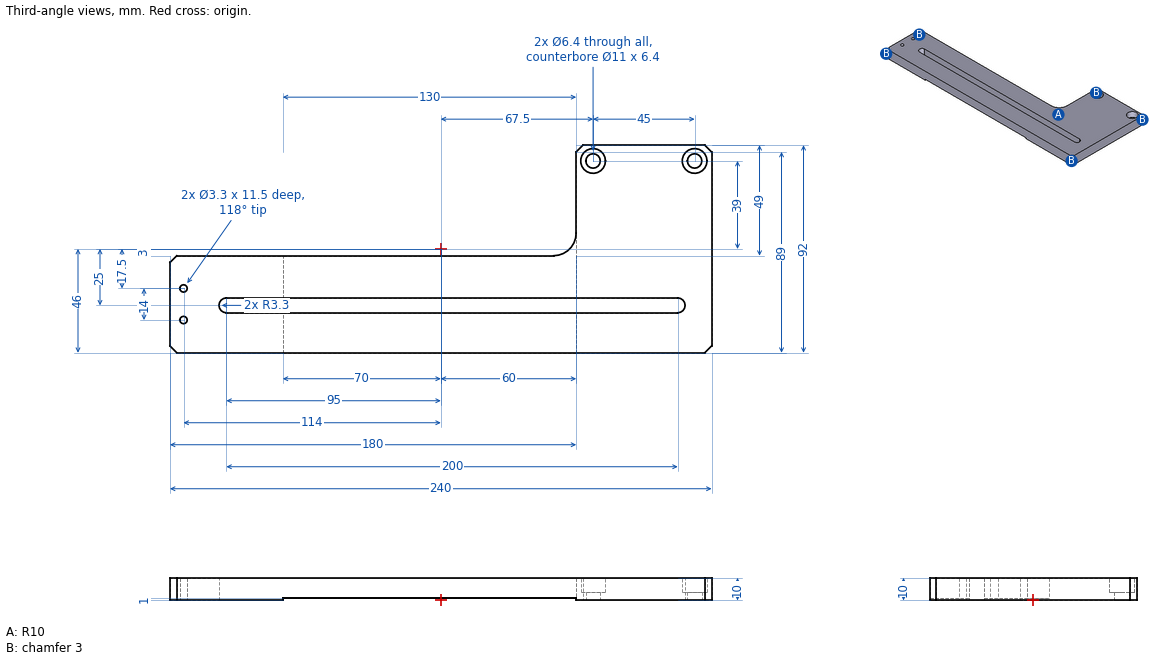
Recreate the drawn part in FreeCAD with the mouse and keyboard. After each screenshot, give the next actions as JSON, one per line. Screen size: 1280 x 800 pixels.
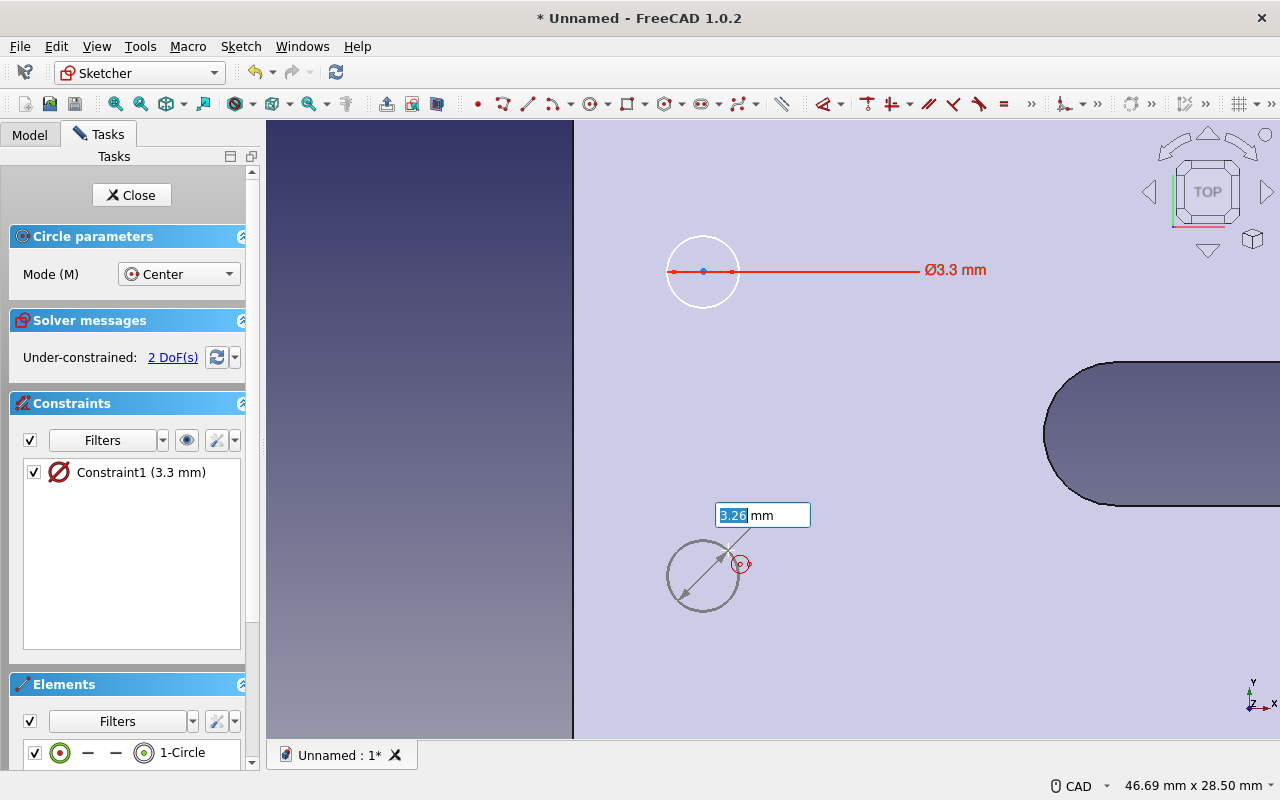
{"action": "type", "text": "3.3"}
{"action": "key", "text": "Return"}
{"action": "key", "text": "Escape"}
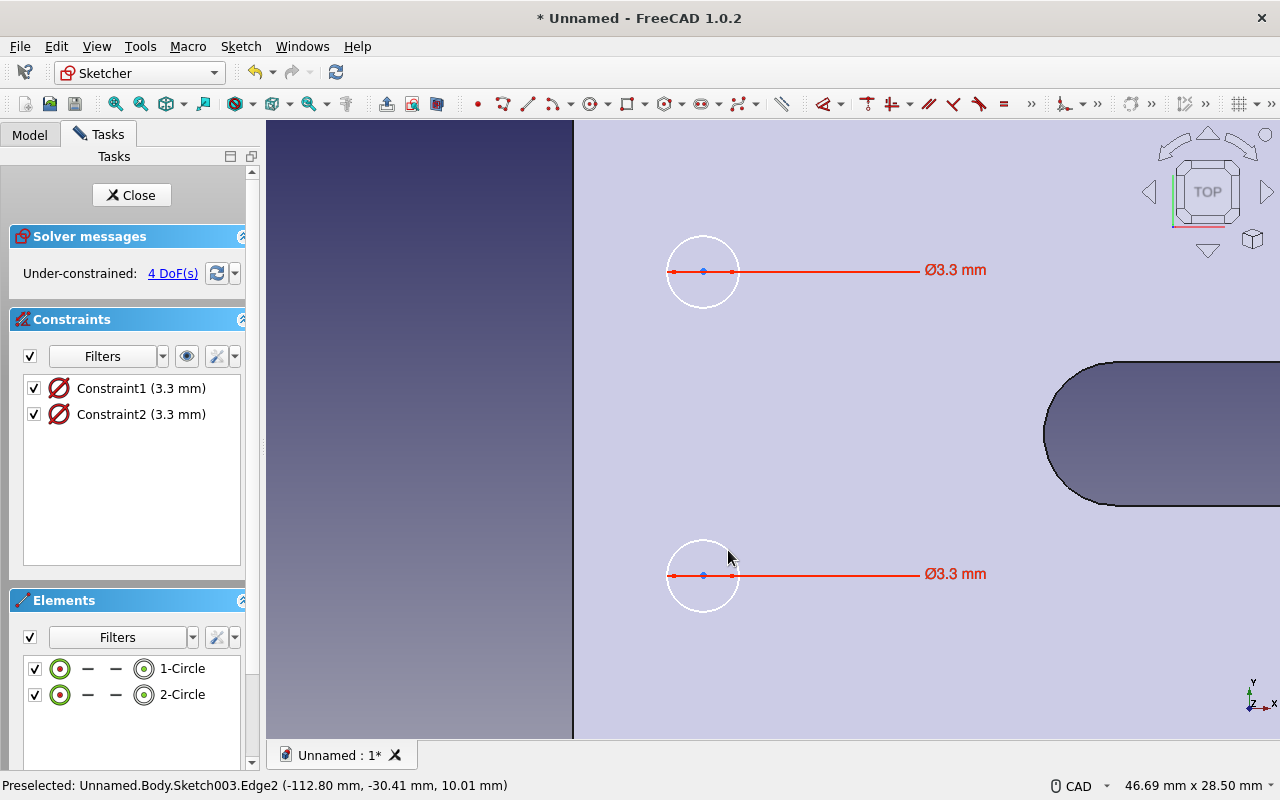
{"action": "left_click", "coordinate": [703, 272]}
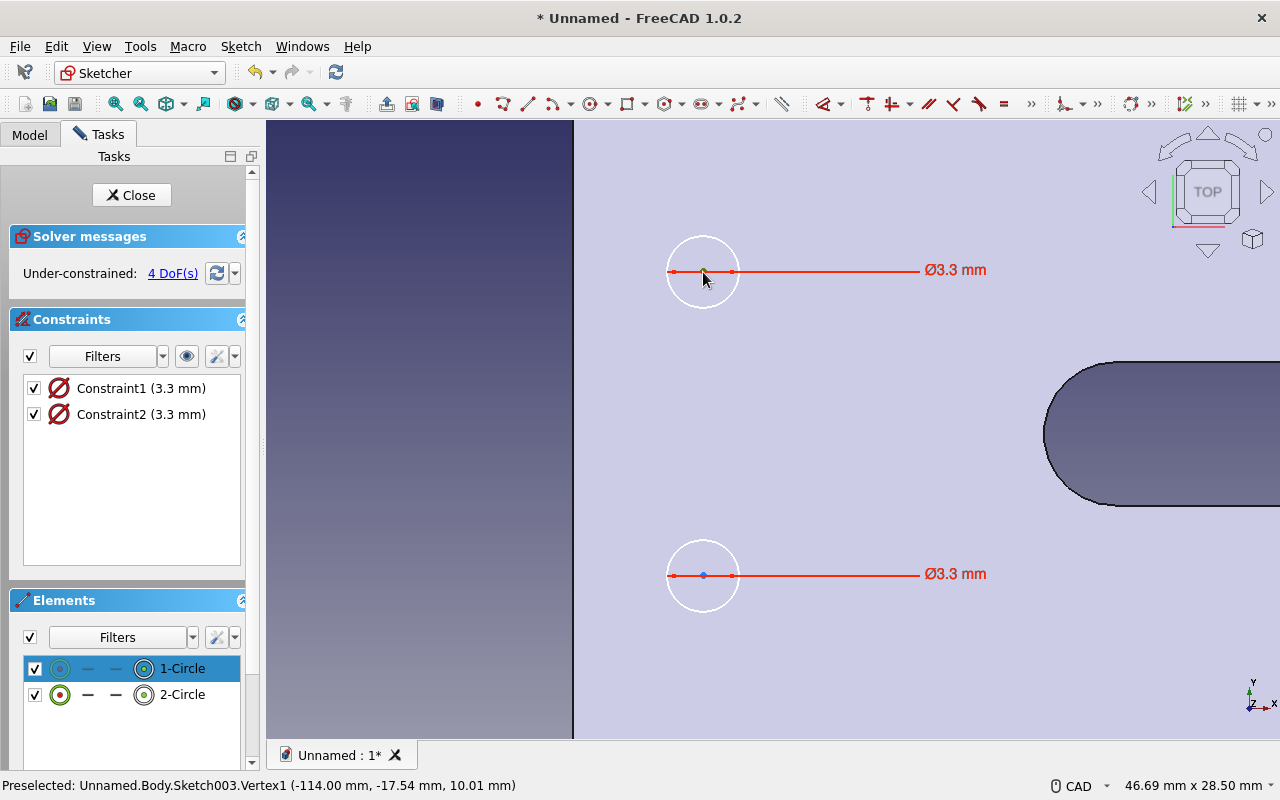
{"action": "left_click", "coordinate": [840, 104]}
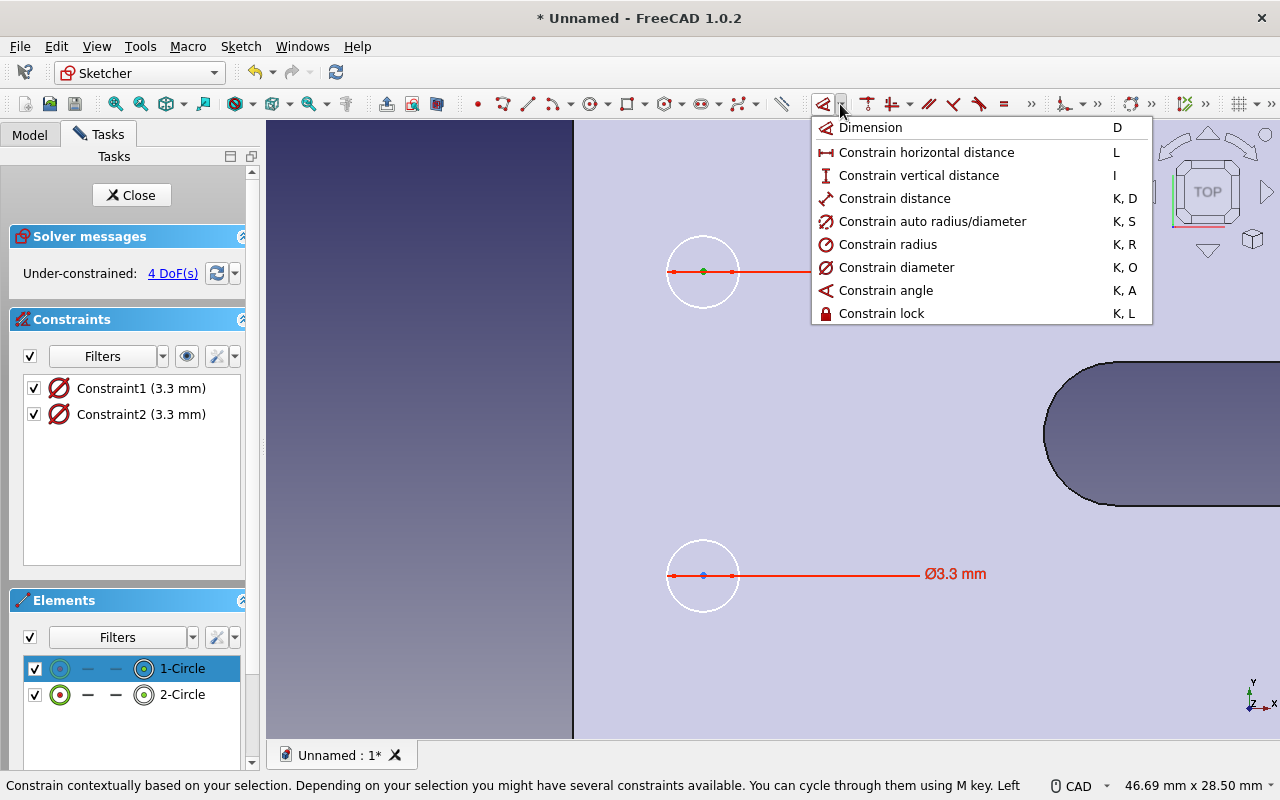
{"action": "left_click", "coordinate": [982, 152]}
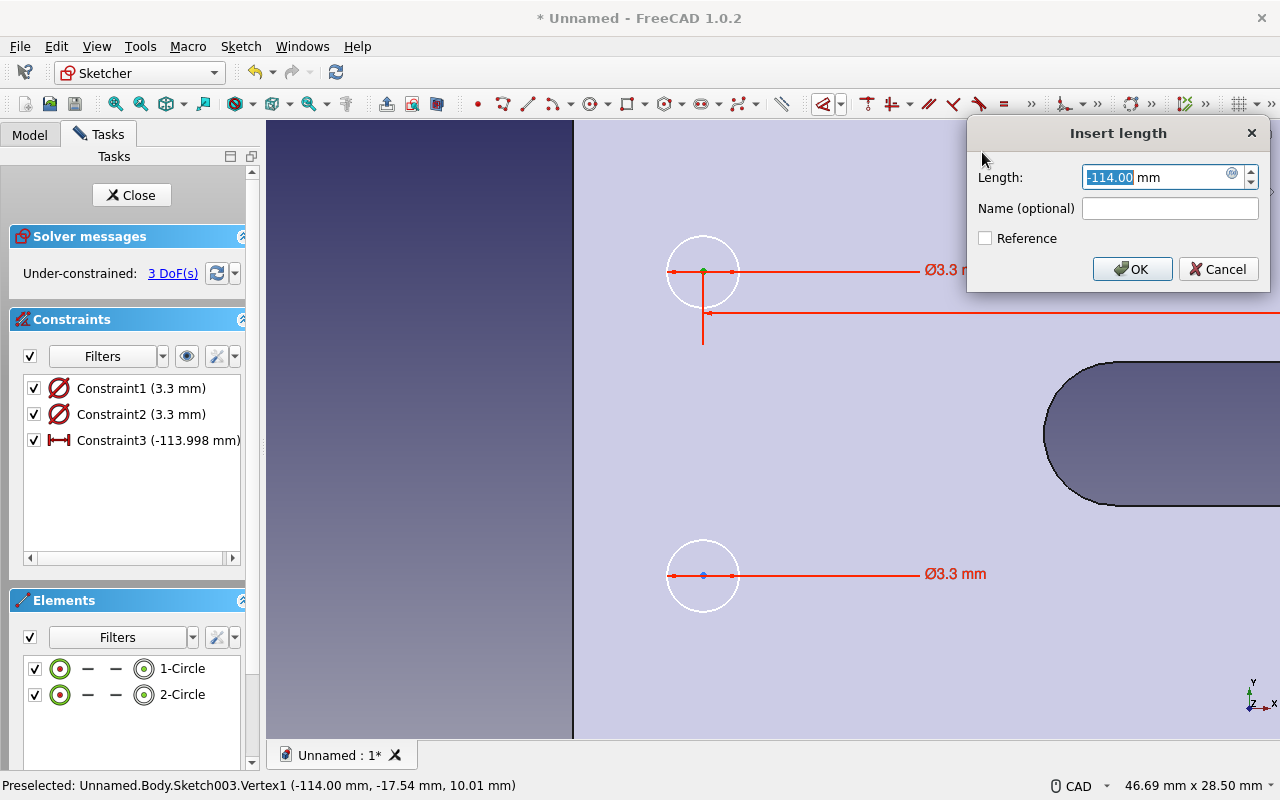
{"action": "type", "text": "-114"}
{"action": "key", "text": "Return"}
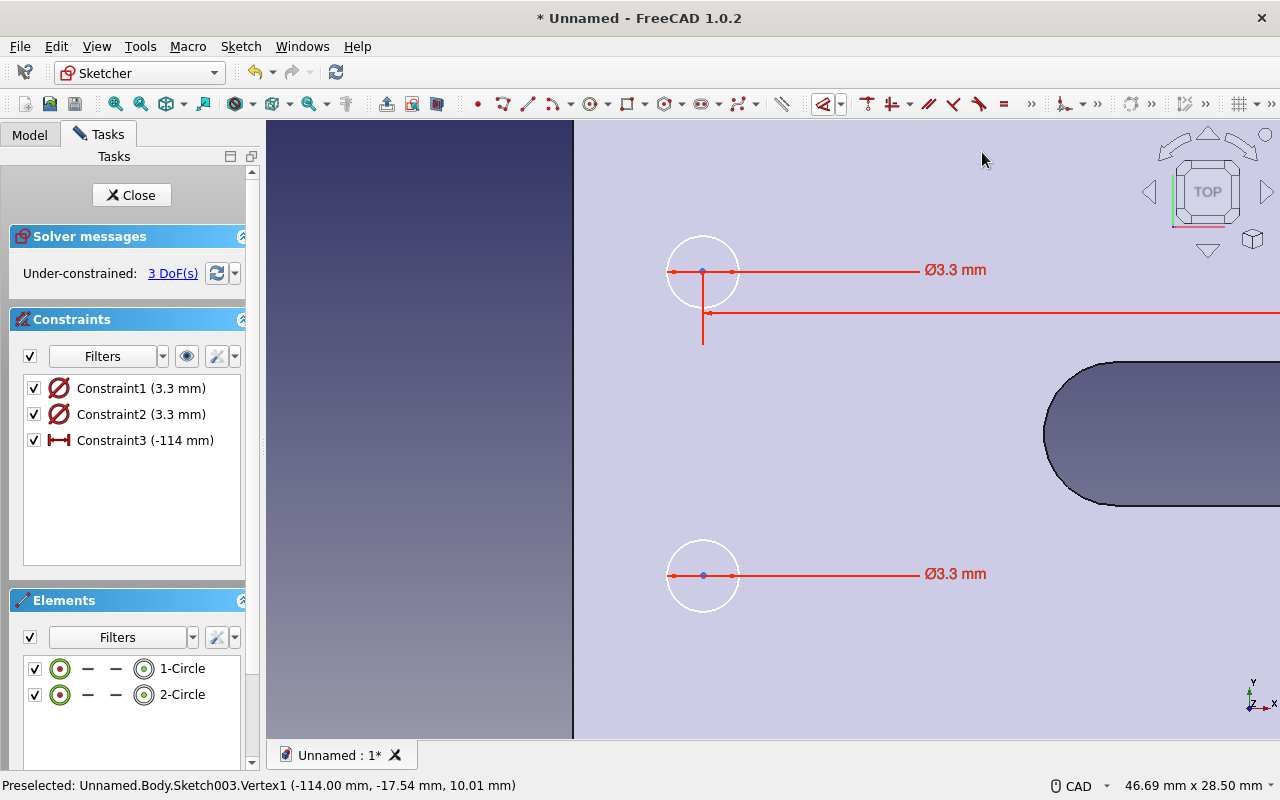
{"action": "left_click", "coordinate": [703, 576]}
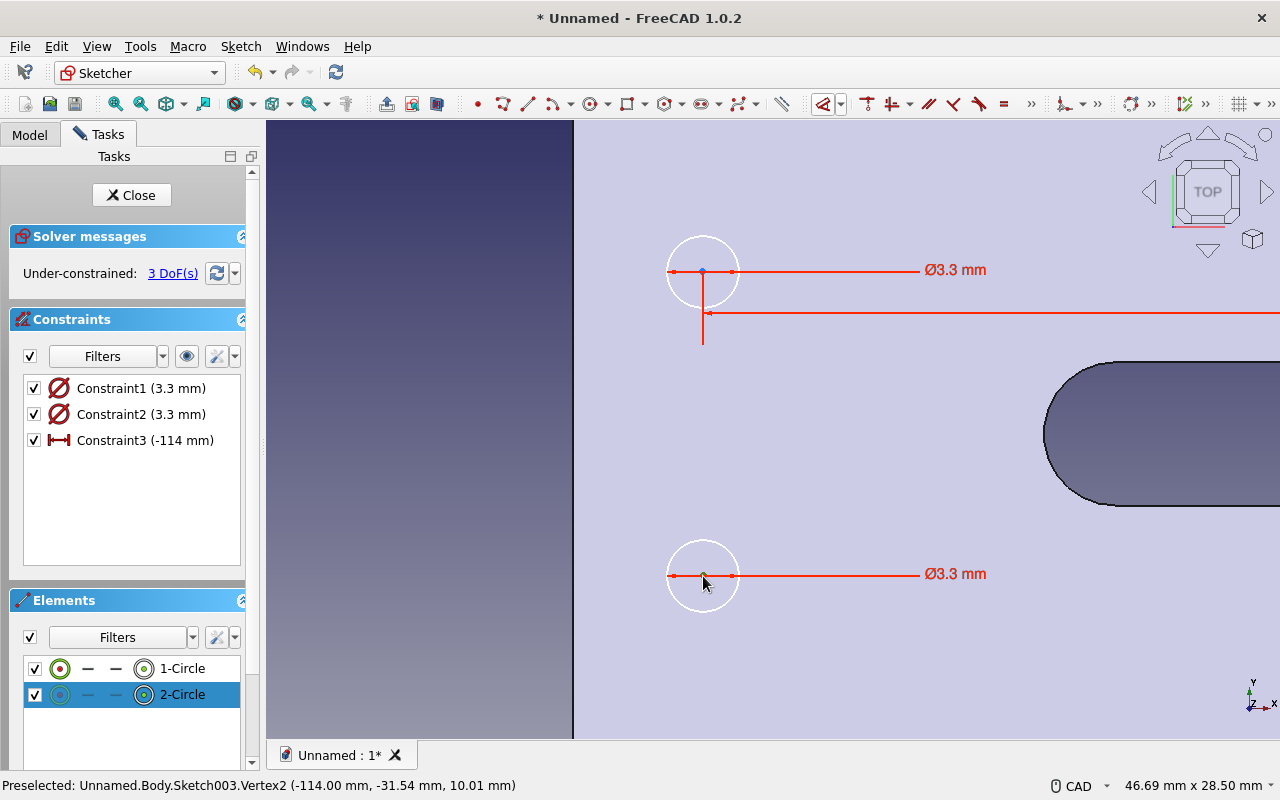
{"action": "key", "text": "l"}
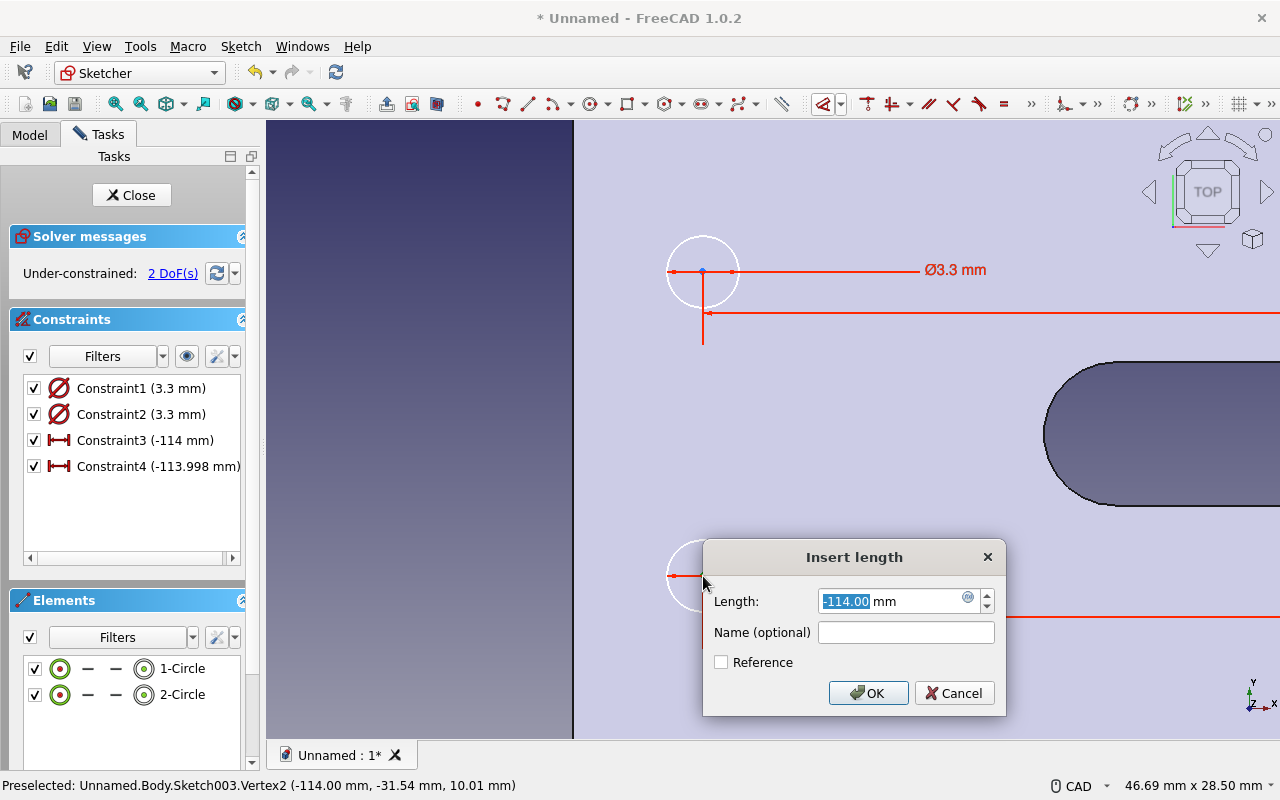
{"action": "type", "text": "-114"}
{"action": "key", "text": "Return"}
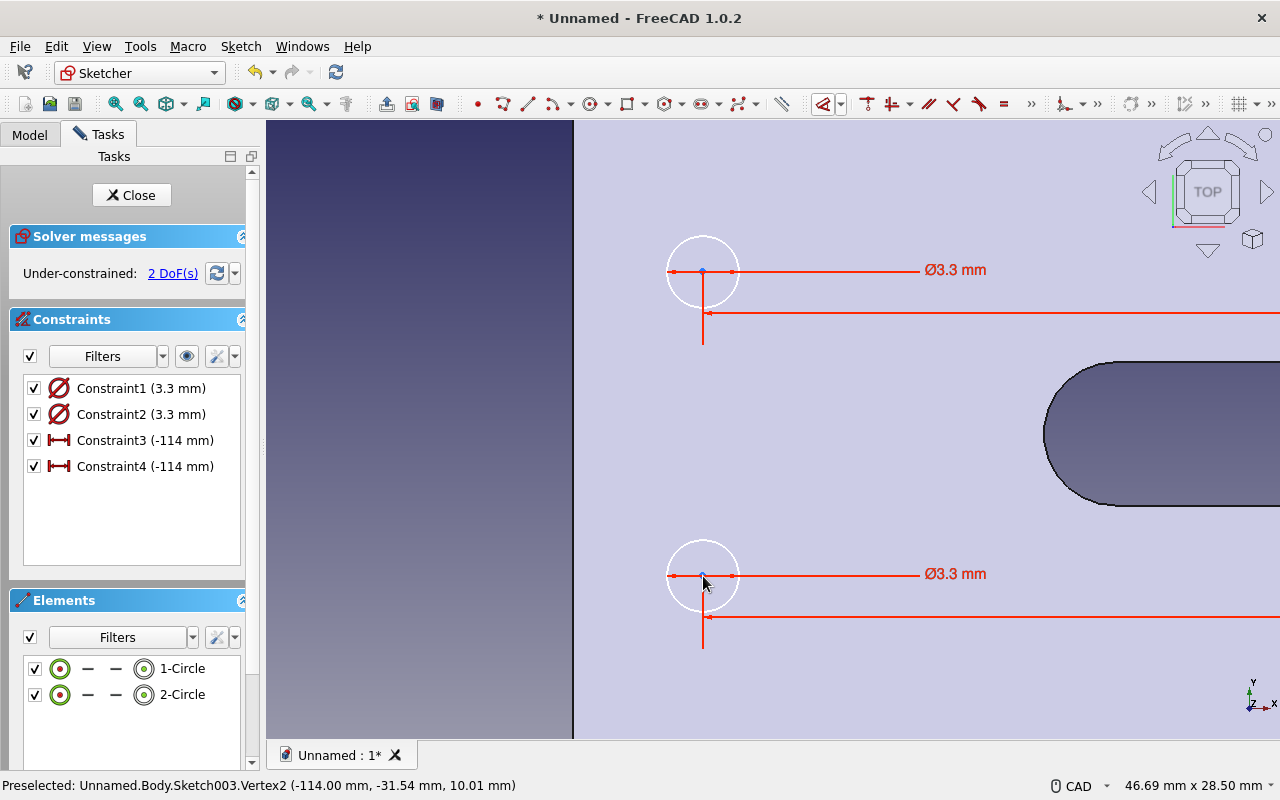
{"action": "left_click", "coordinate": [703, 272]}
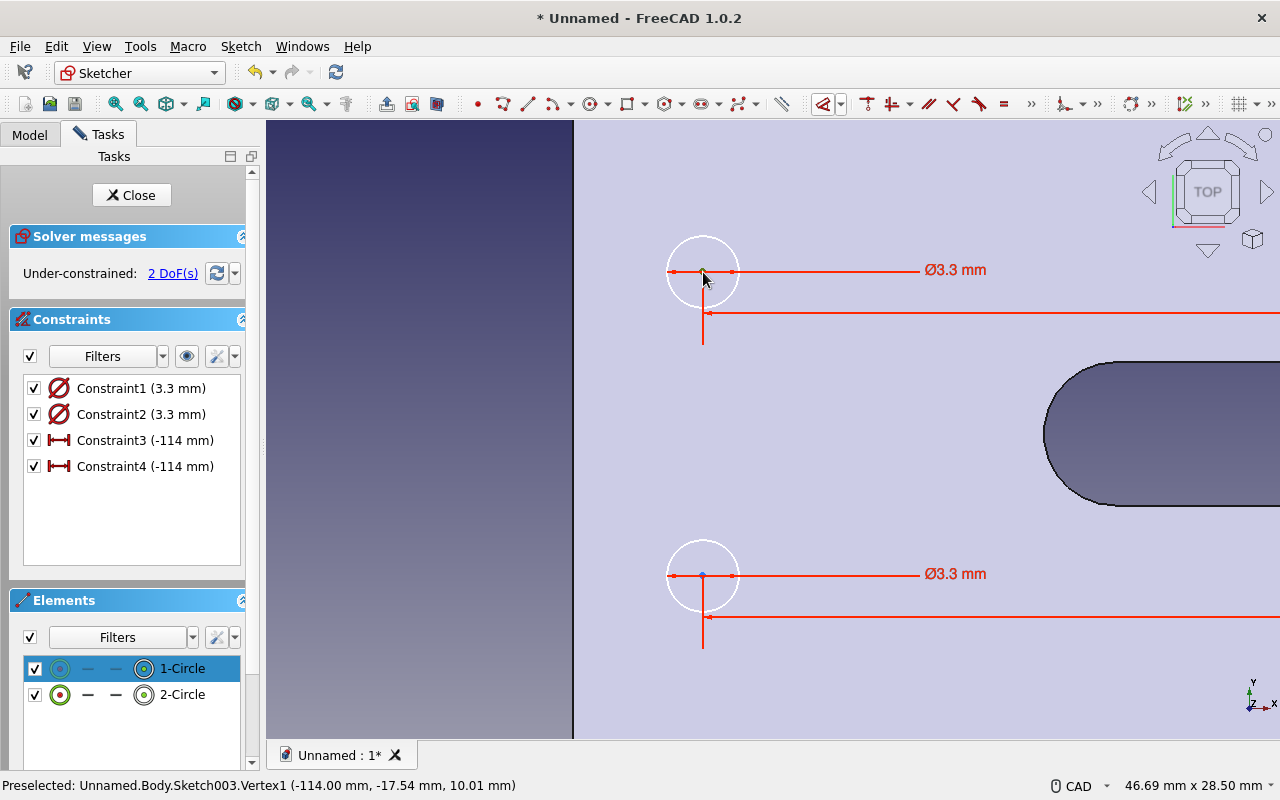
{"action": "left_click", "coordinate": [703, 576]}